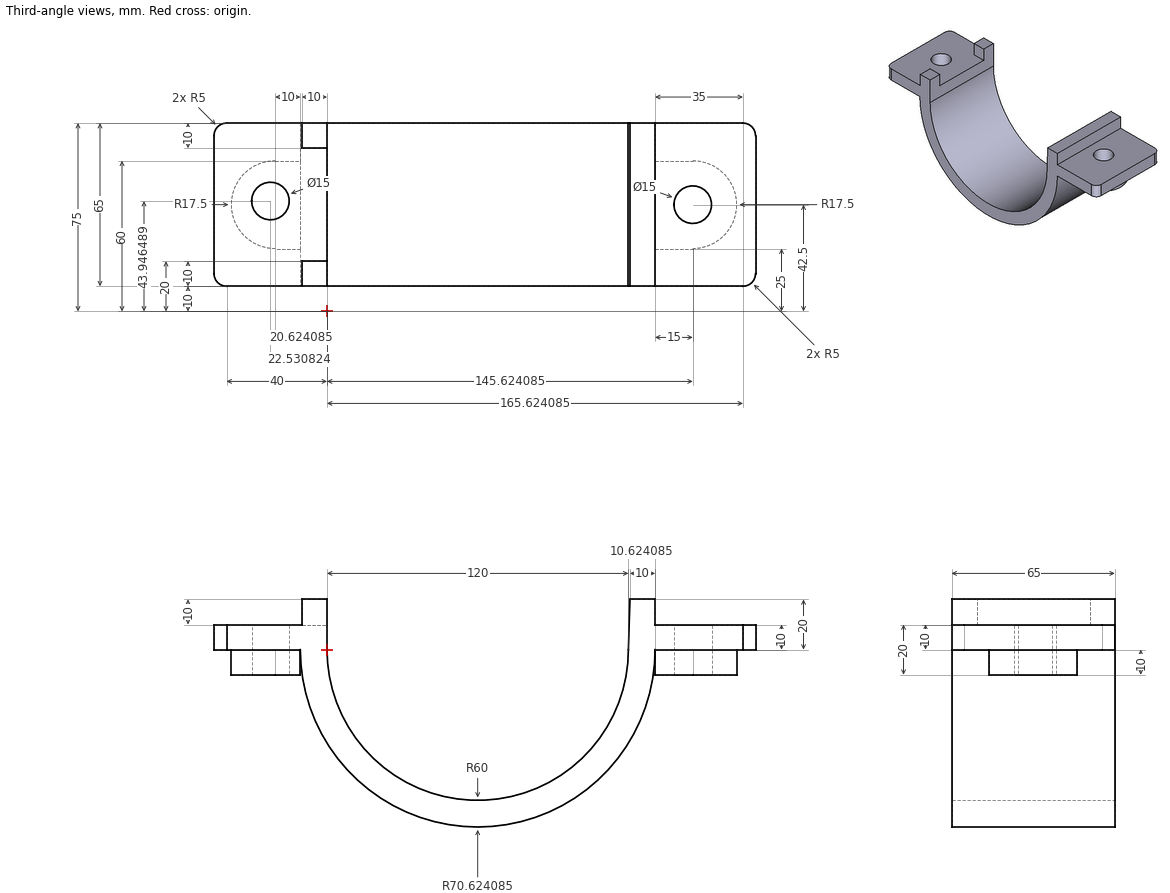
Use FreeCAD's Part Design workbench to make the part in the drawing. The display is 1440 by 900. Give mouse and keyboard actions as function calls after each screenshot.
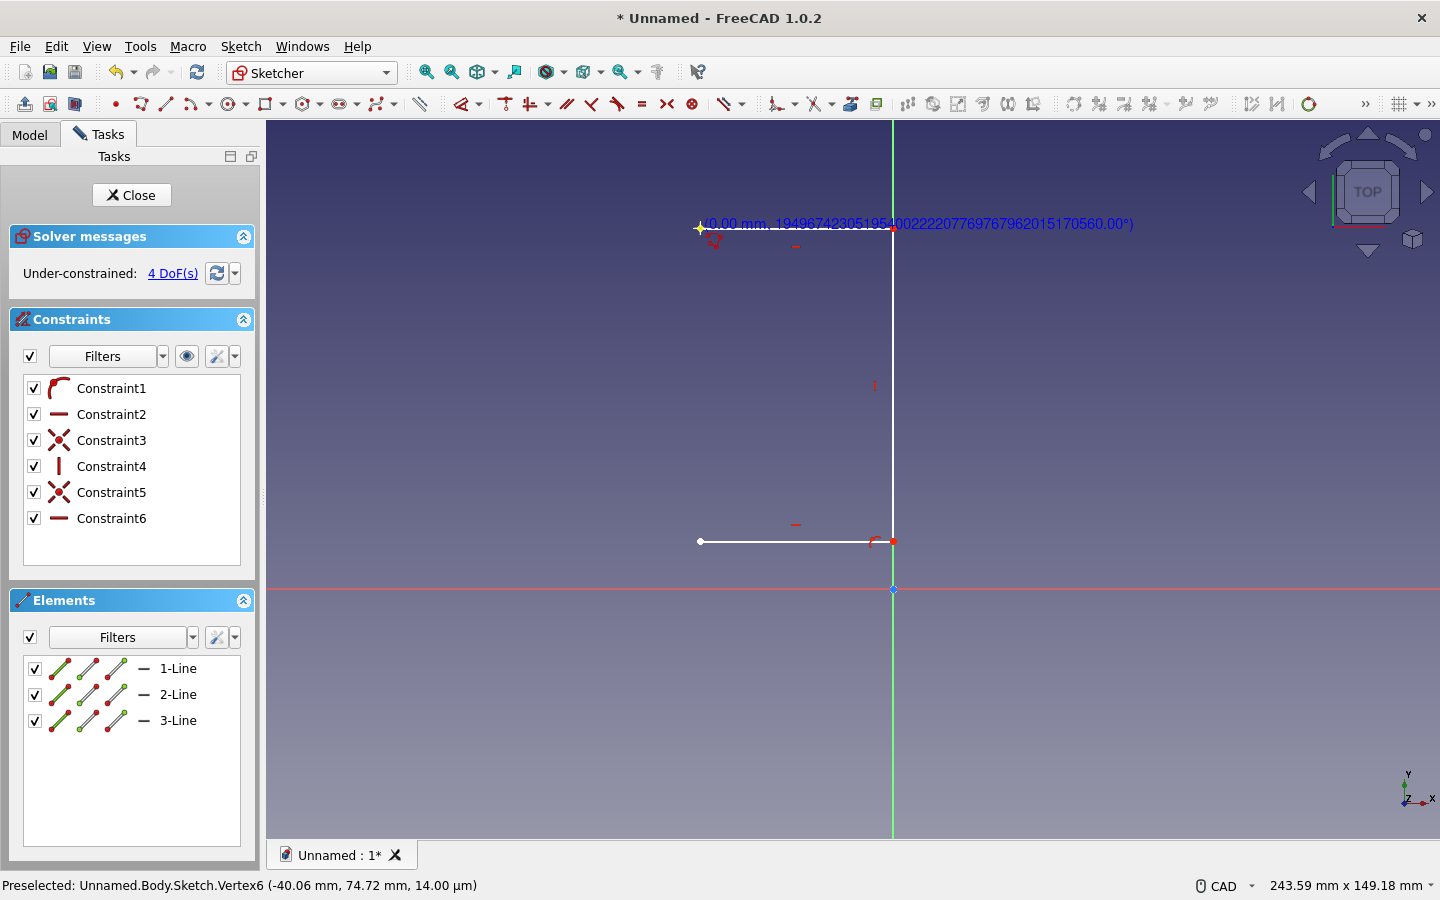
click(166, 104)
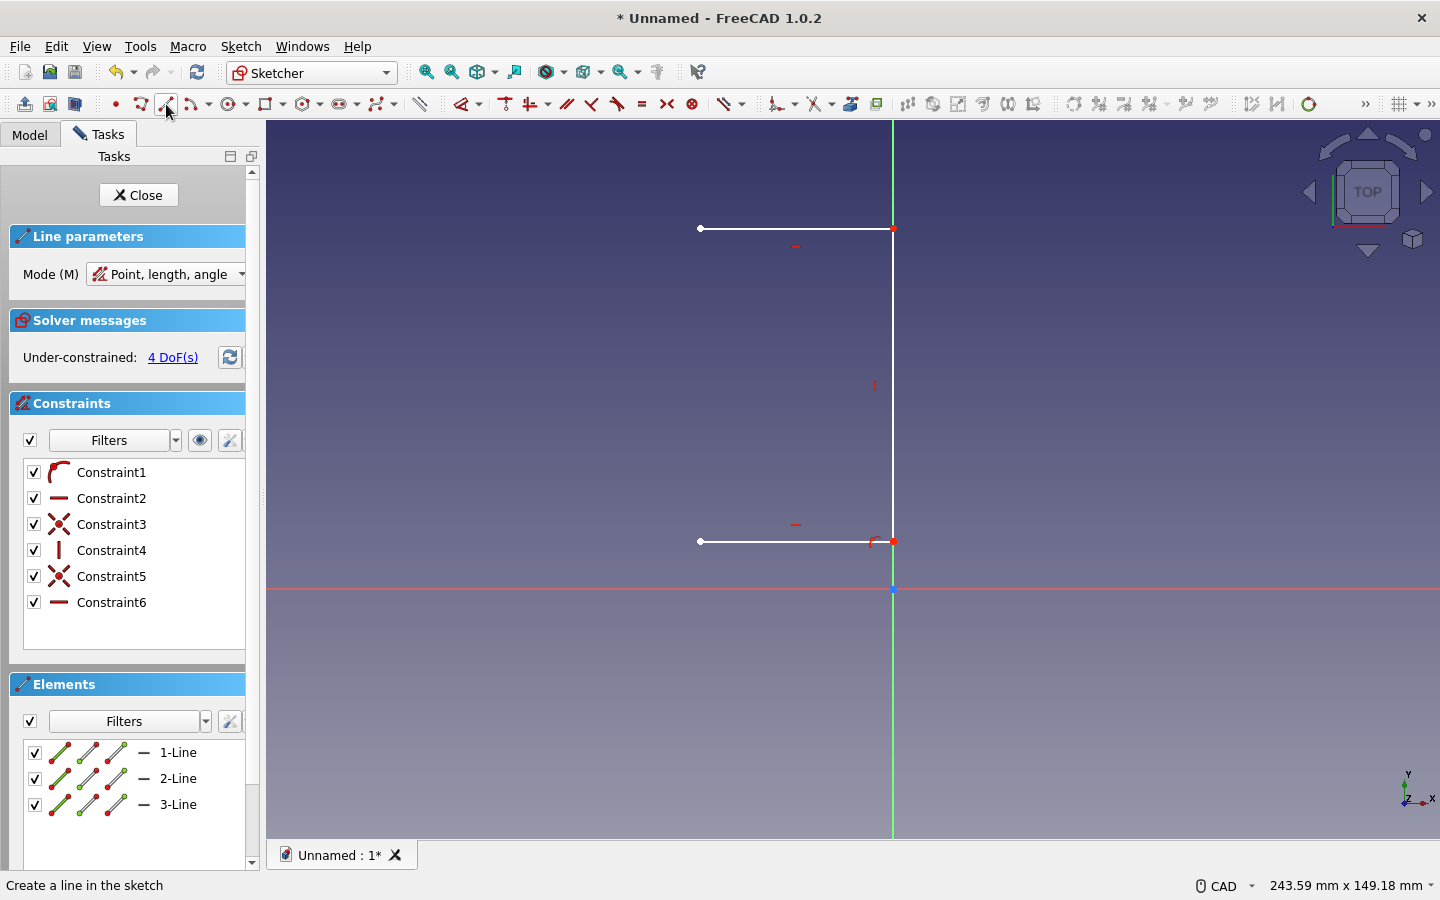
click(676, 252)
click(676, 517)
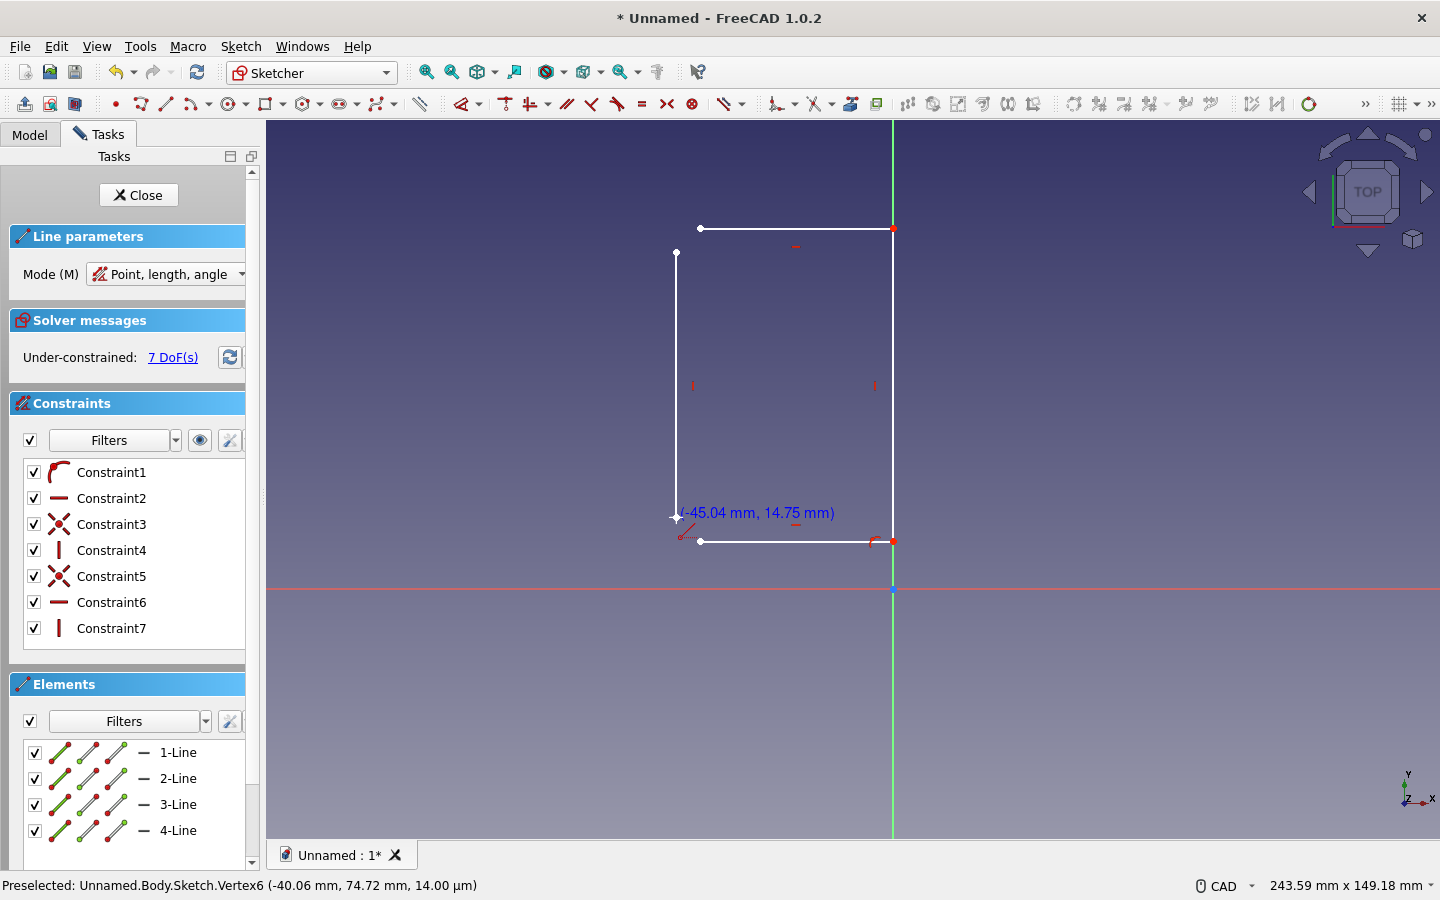
key(g)
key(3)
key(a)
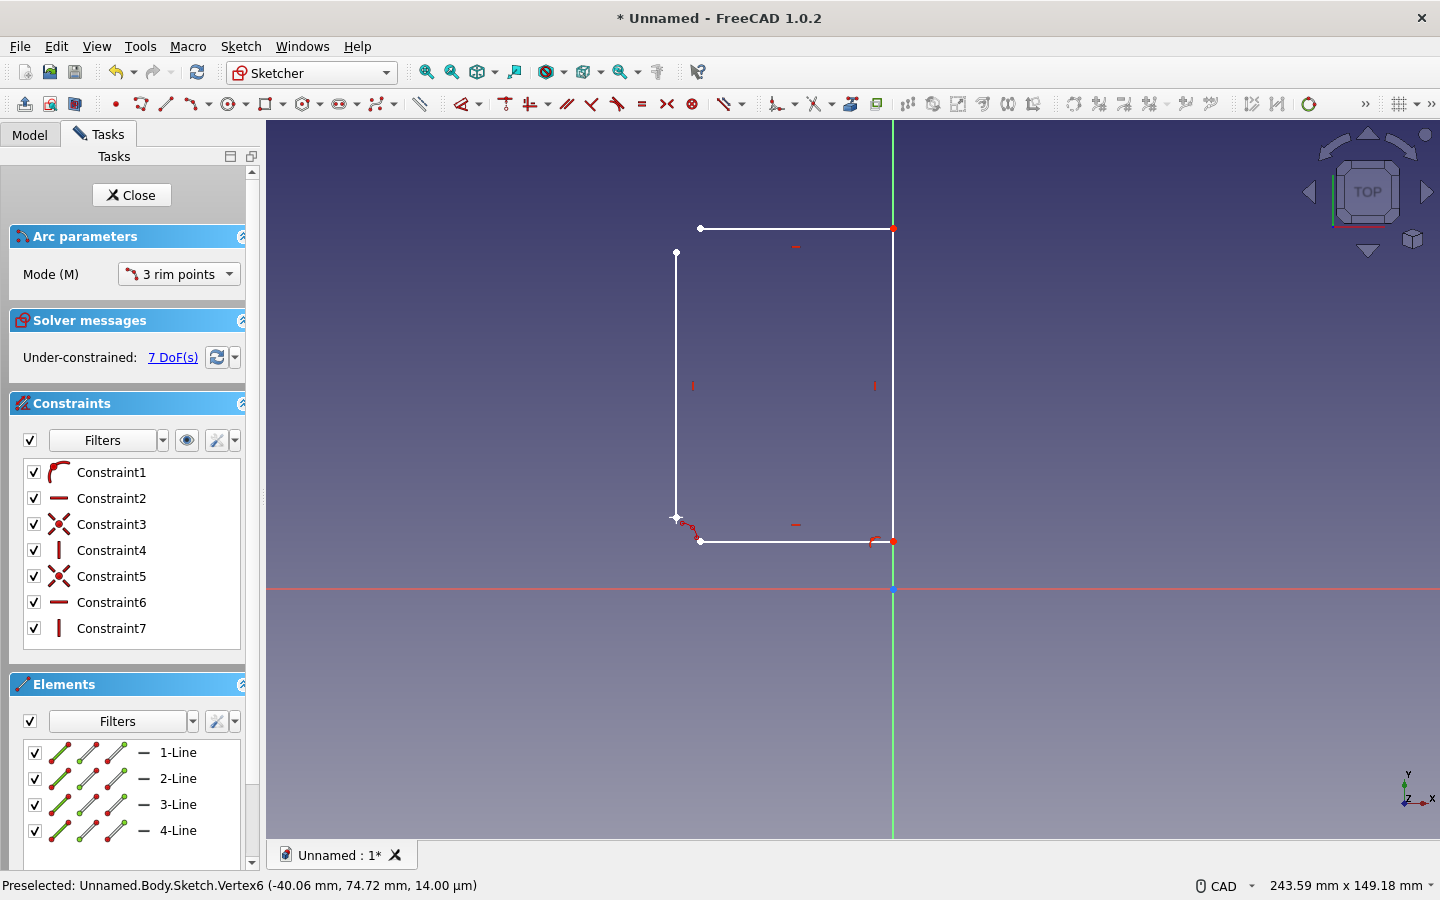
click(700, 229)
click(676, 253)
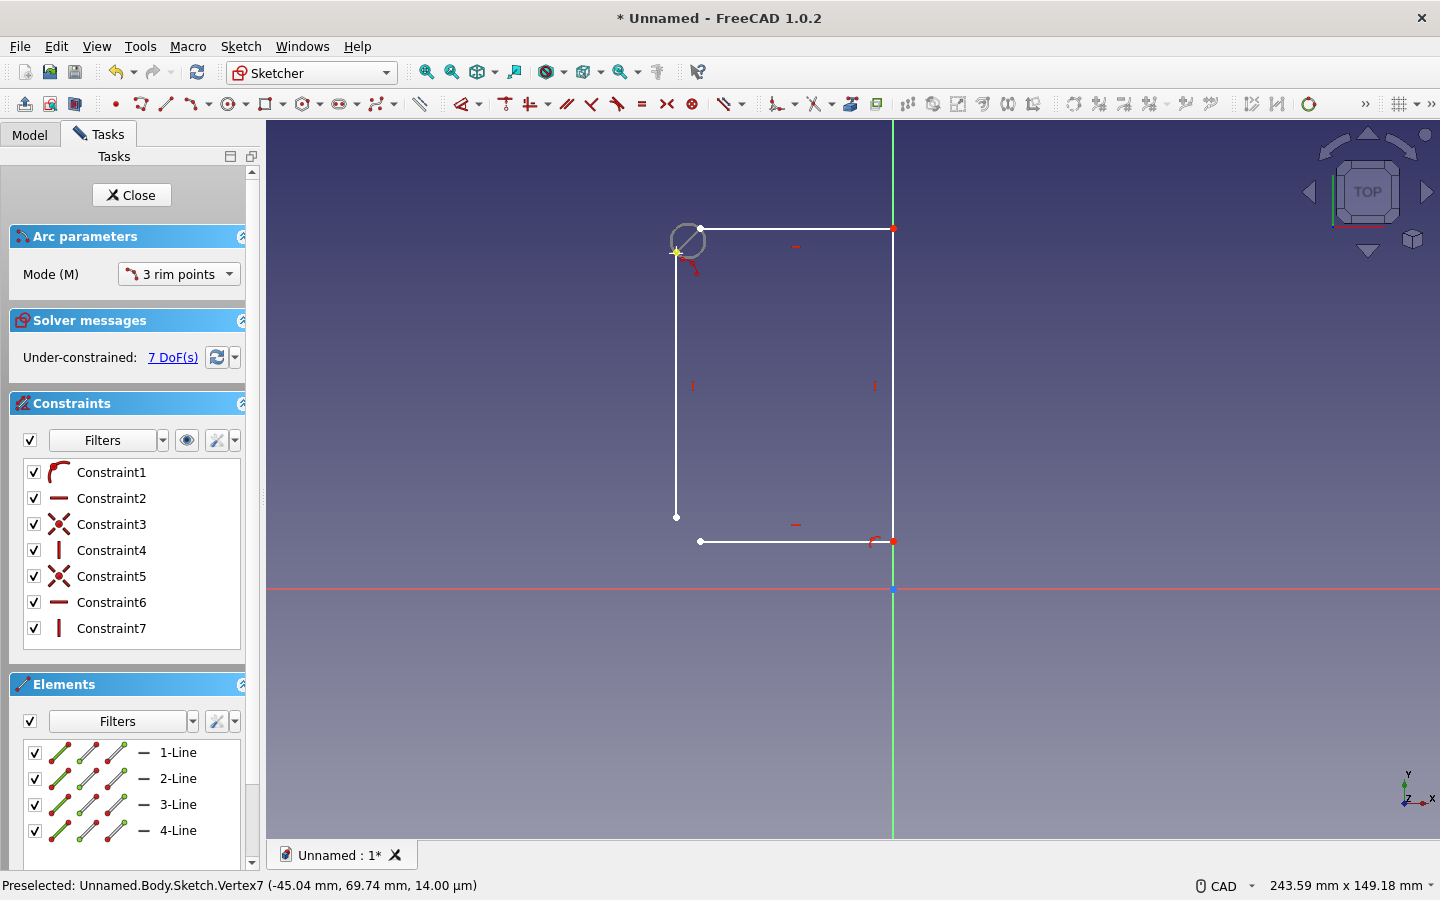
scroll(683, 235, up, 5)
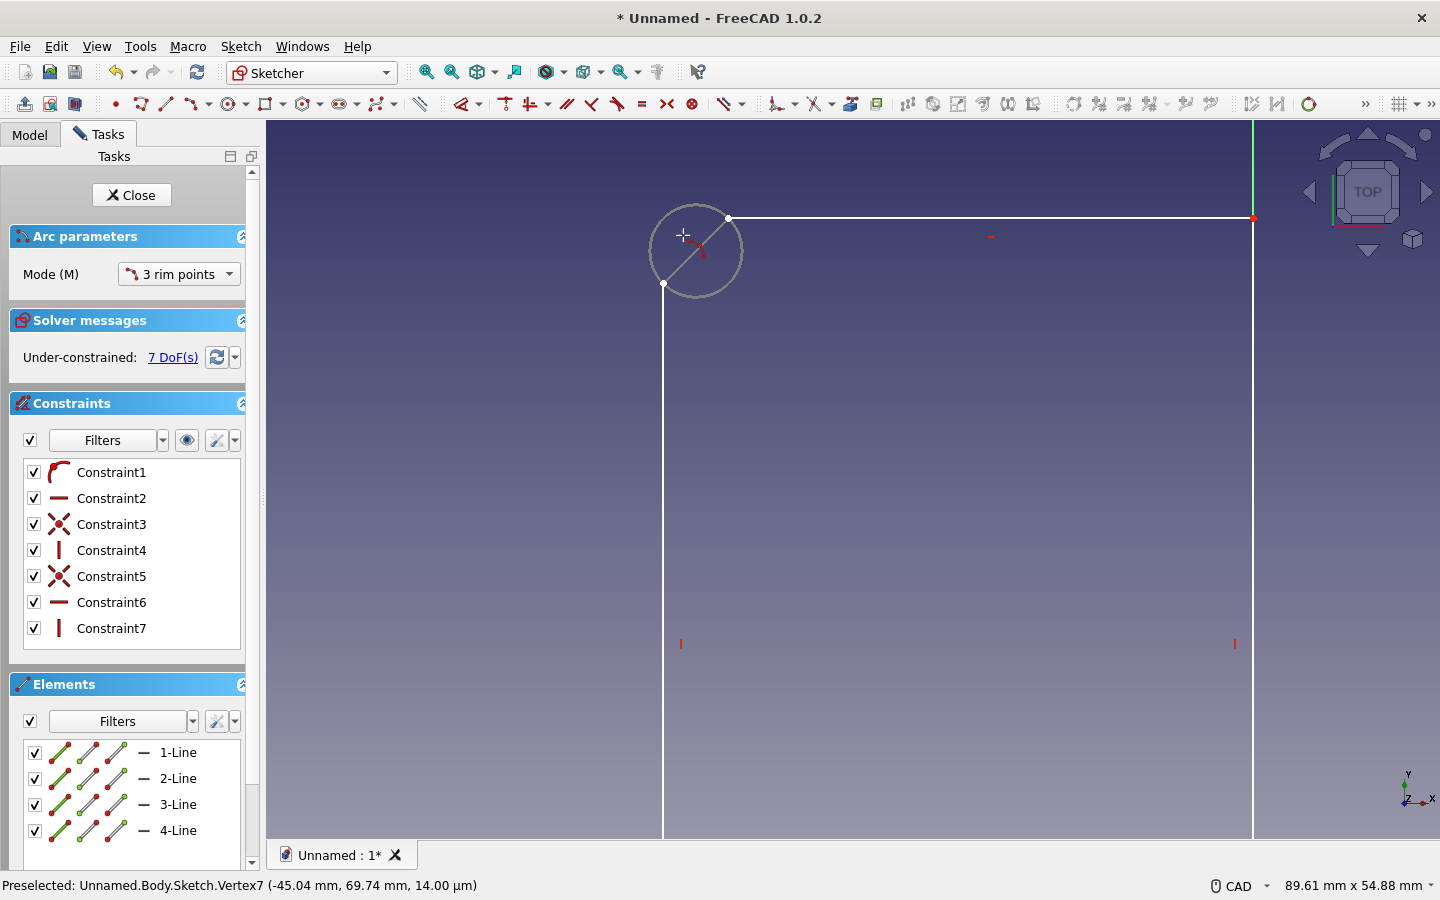
click(683, 234)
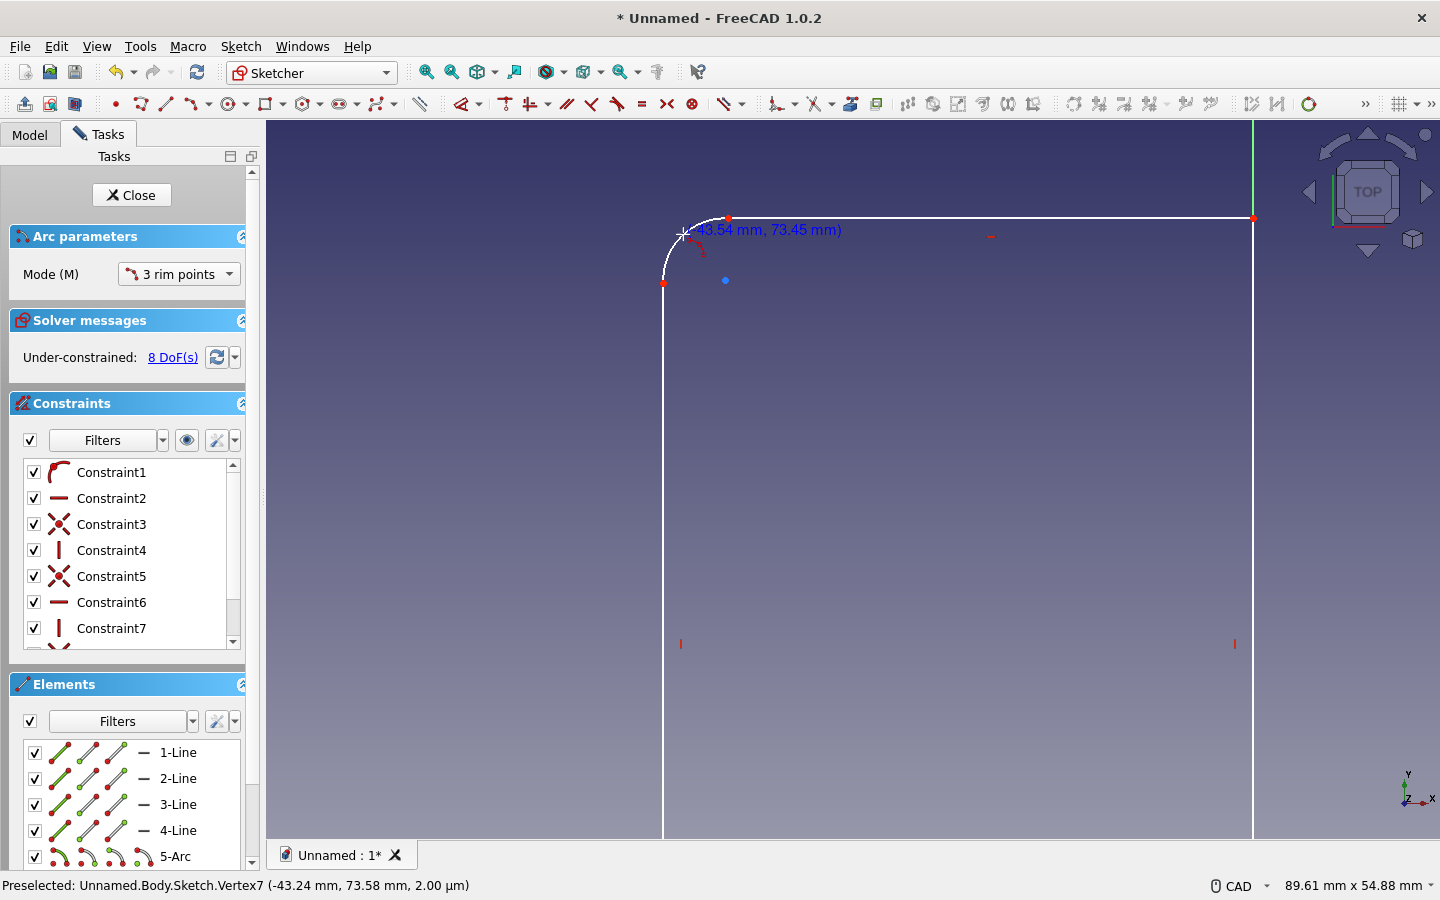
scroll(642, 295, down, 4)